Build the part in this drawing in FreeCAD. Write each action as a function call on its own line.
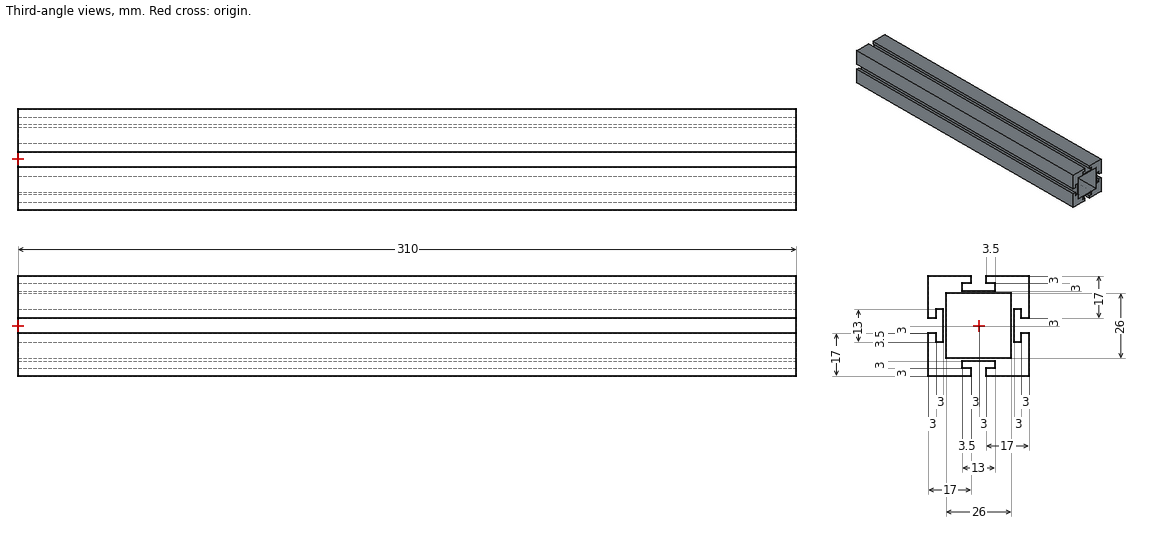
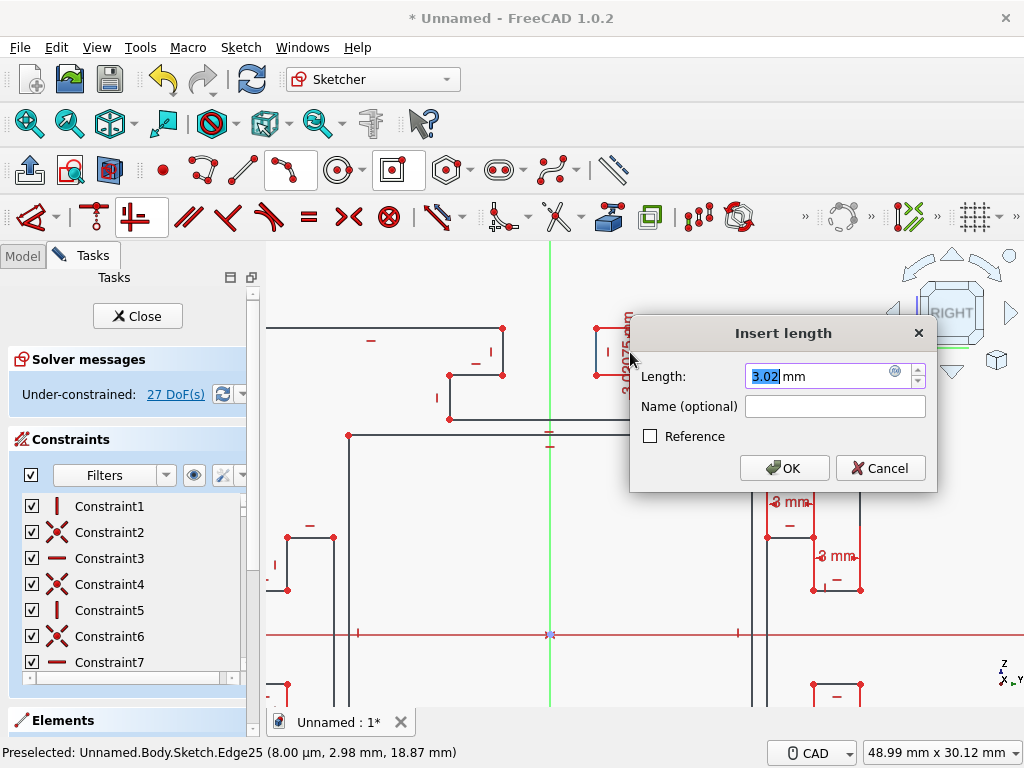
text(3)
key(Return)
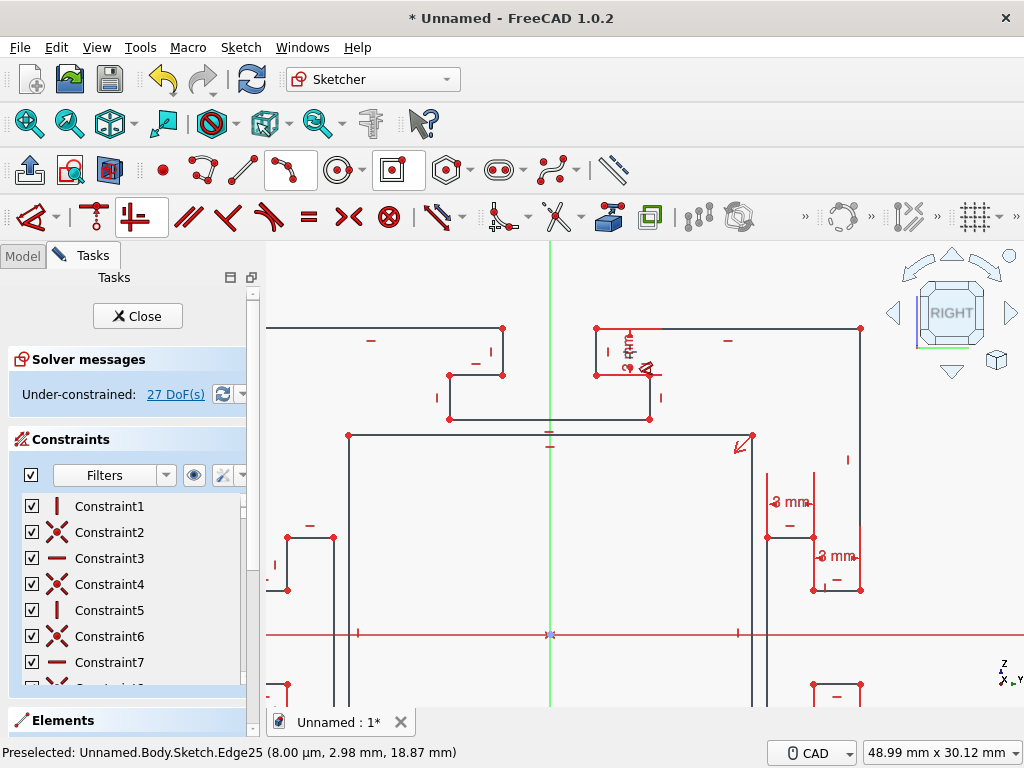
click(650, 388)
click(684, 397)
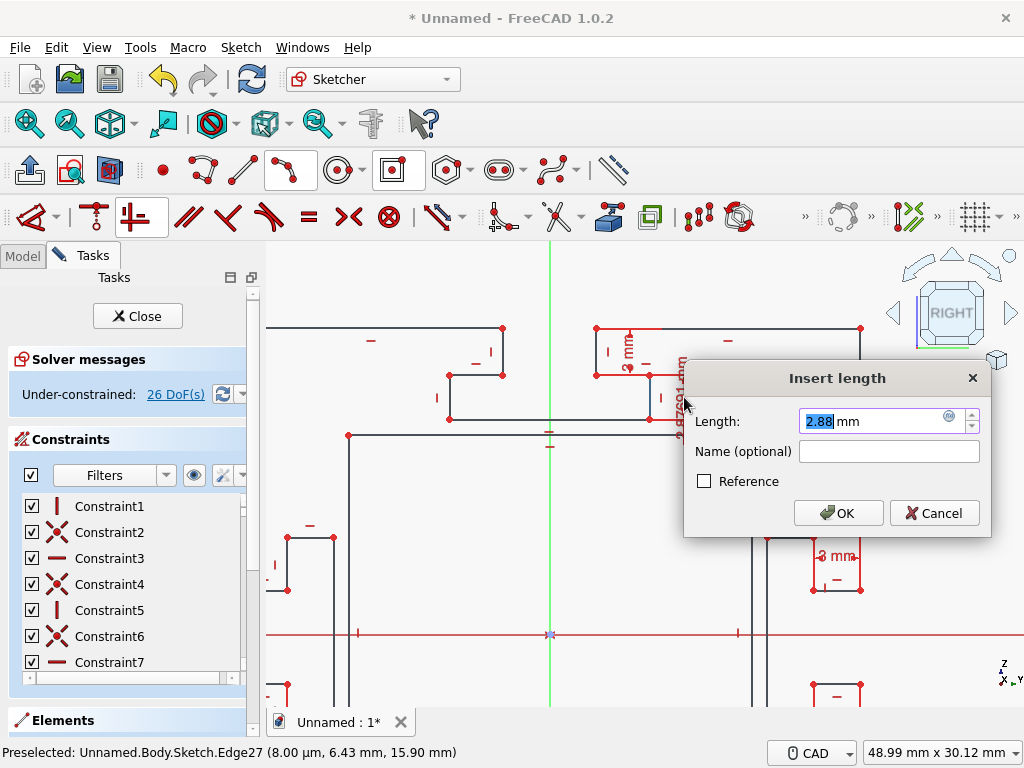
text(3)
key(Return)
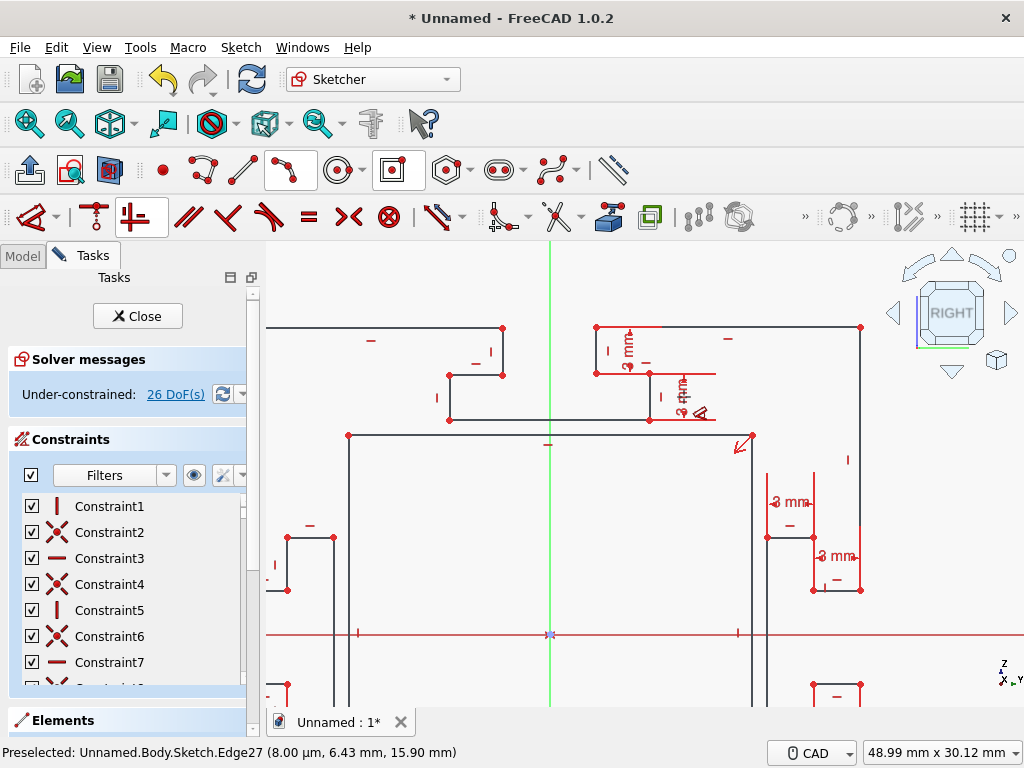
click(450, 407)
click(416, 398)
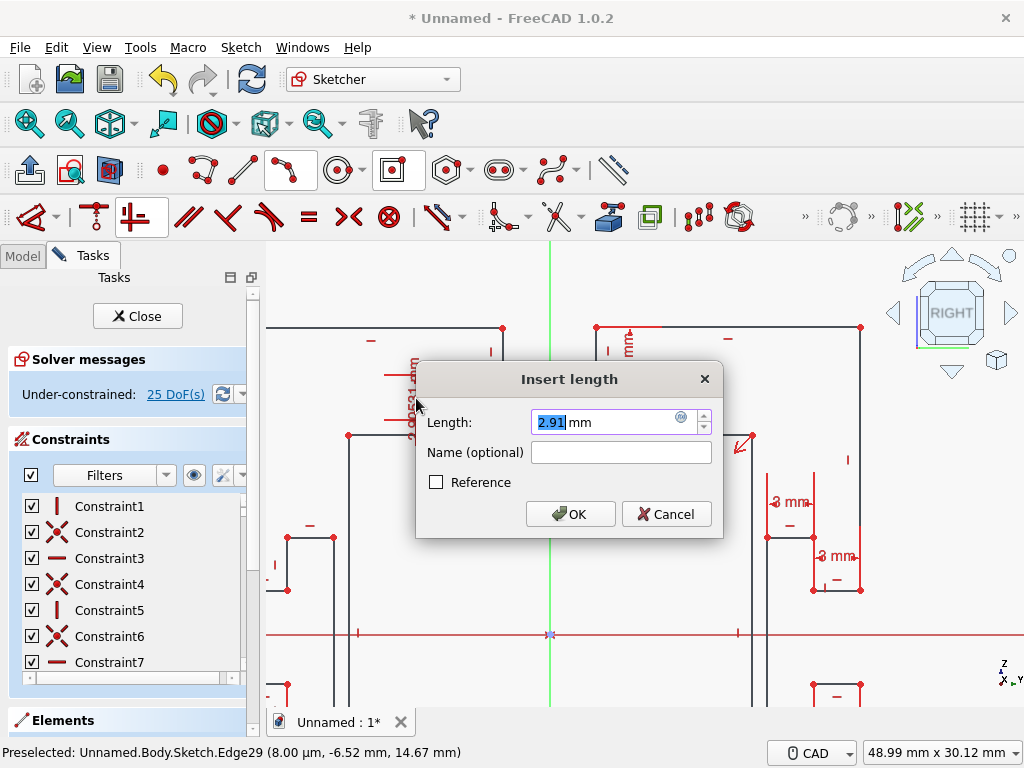
text(3)
key(Return)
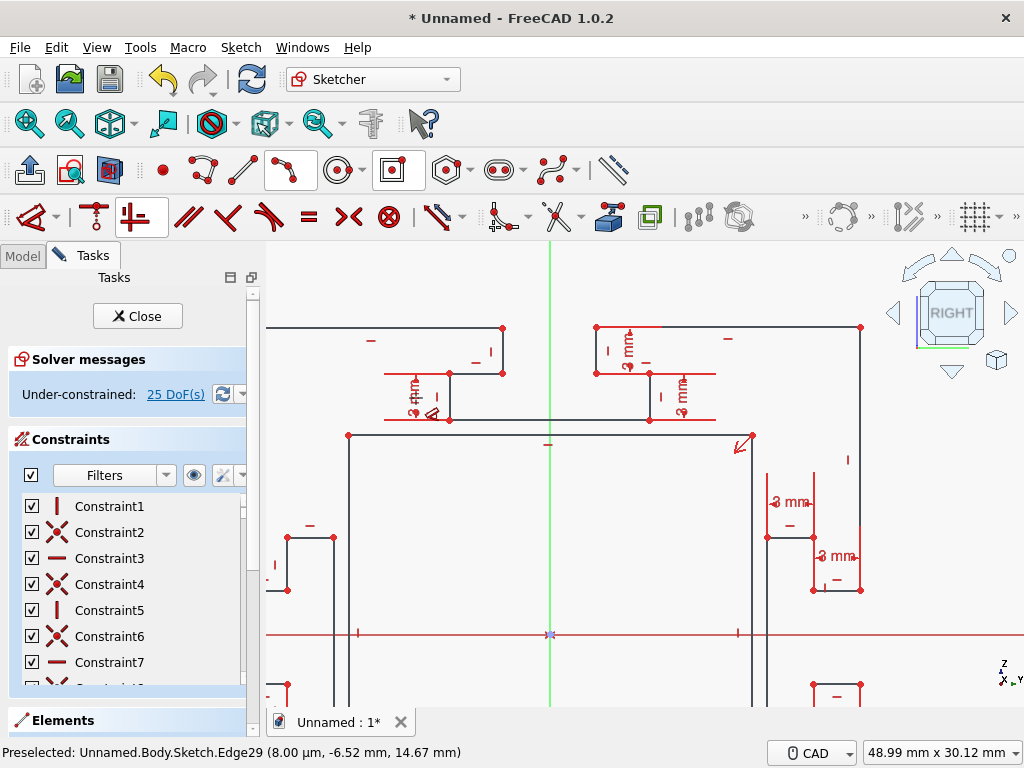
click(503, 360)
click(469, 351)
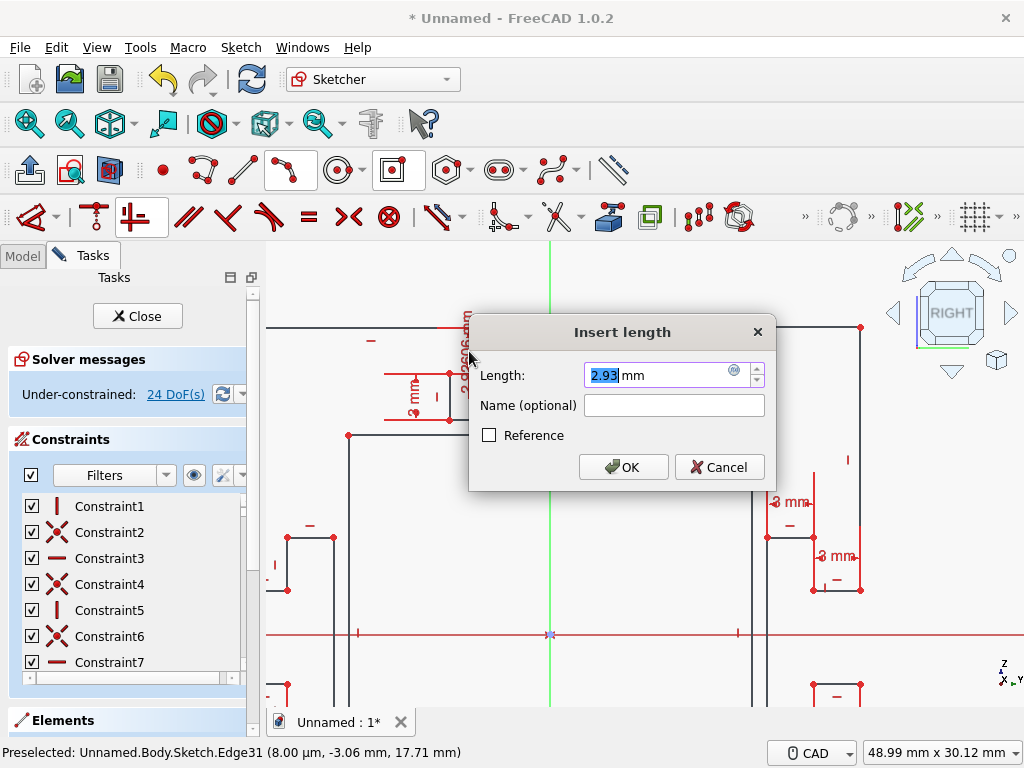
text(3)
key(Return)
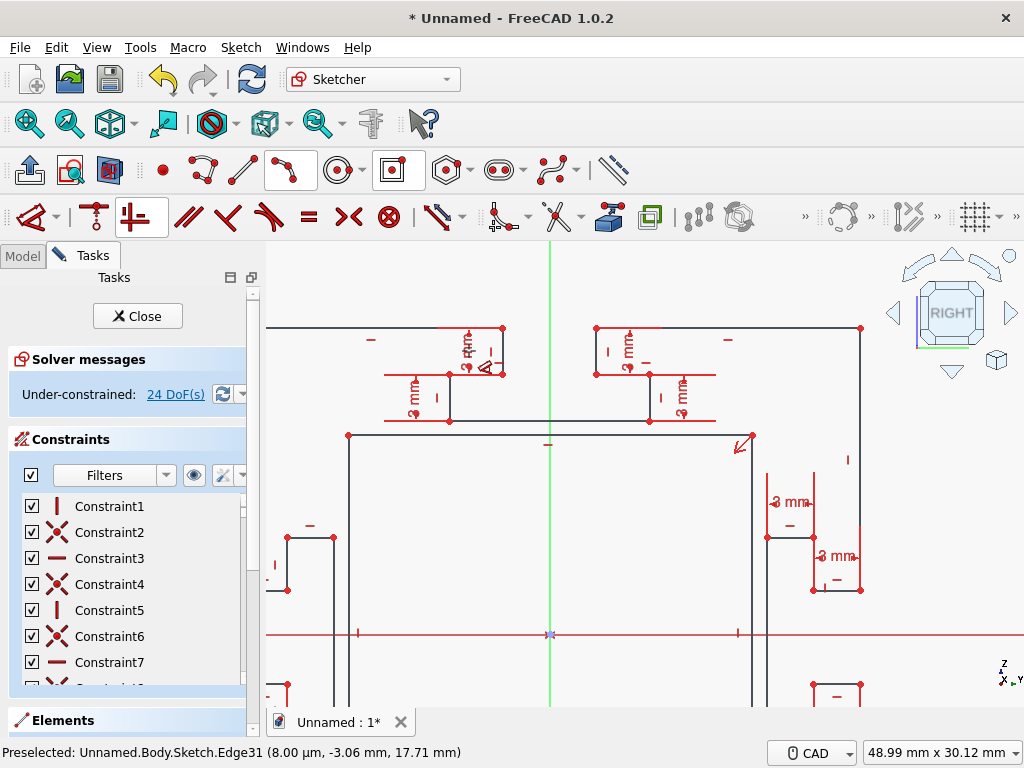
scroll(598, 343, down, 4)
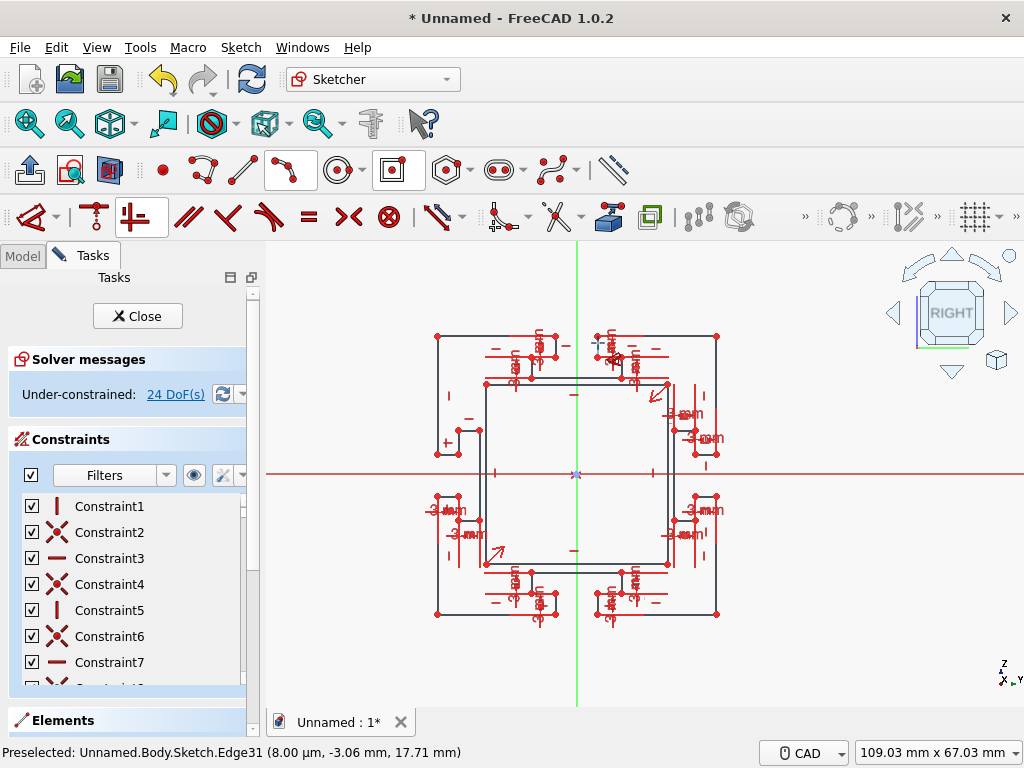
scroll(444, 455, up, 4)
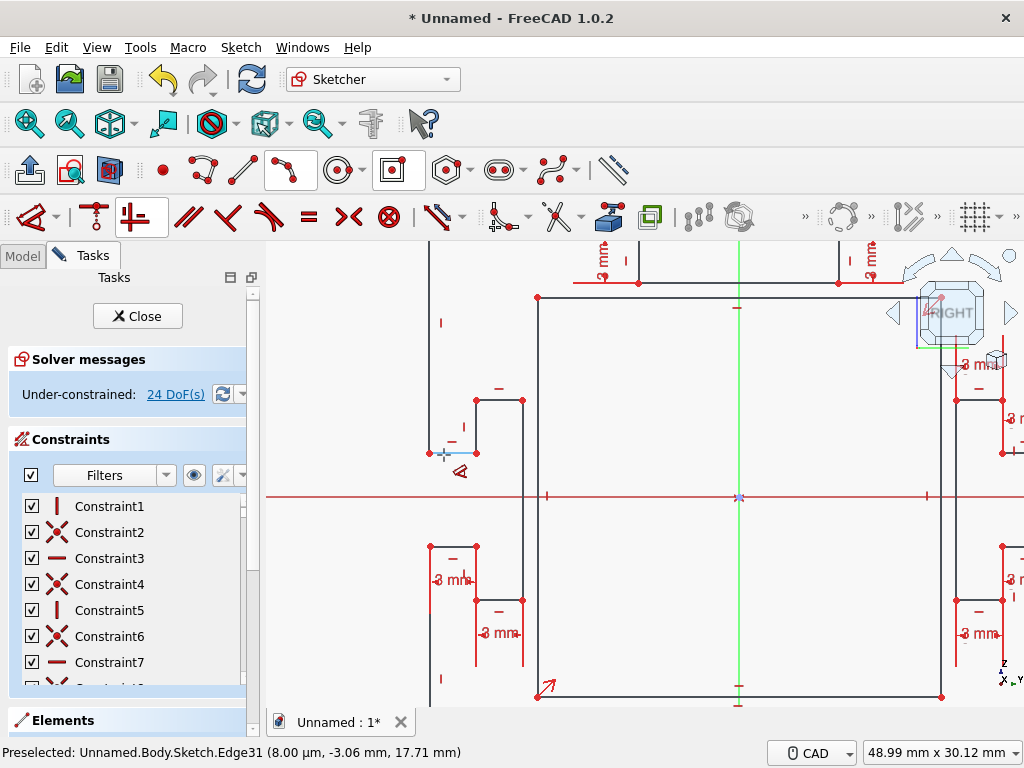
click(443, 453)
click(453, 419)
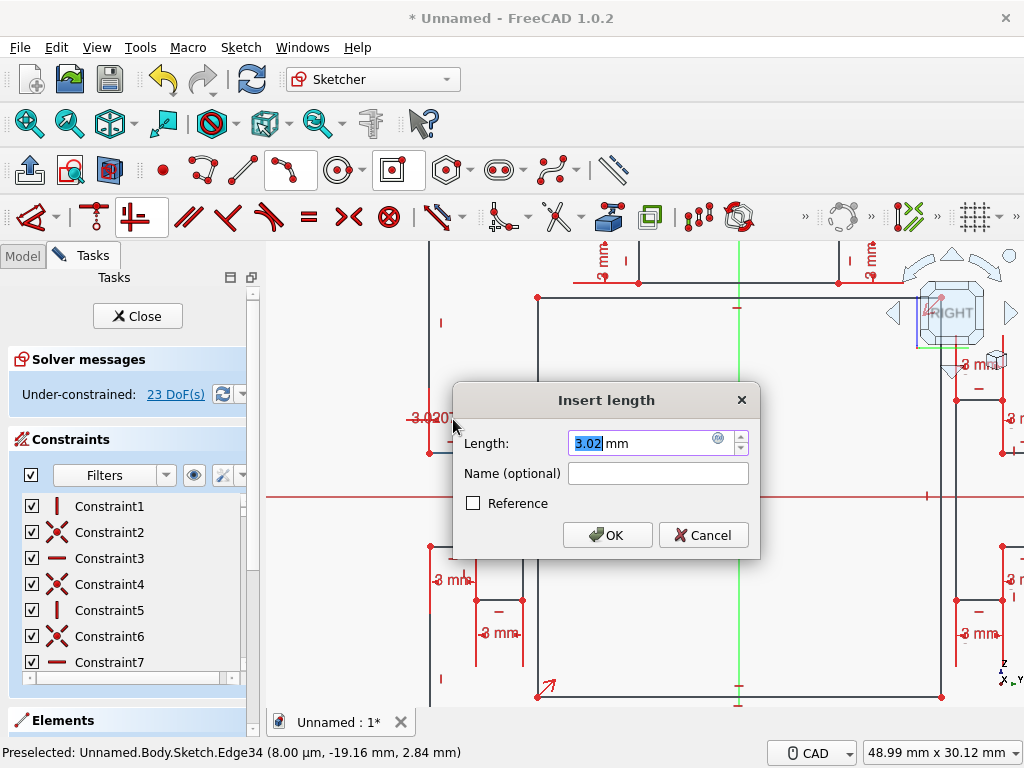
text(3)
key(Return)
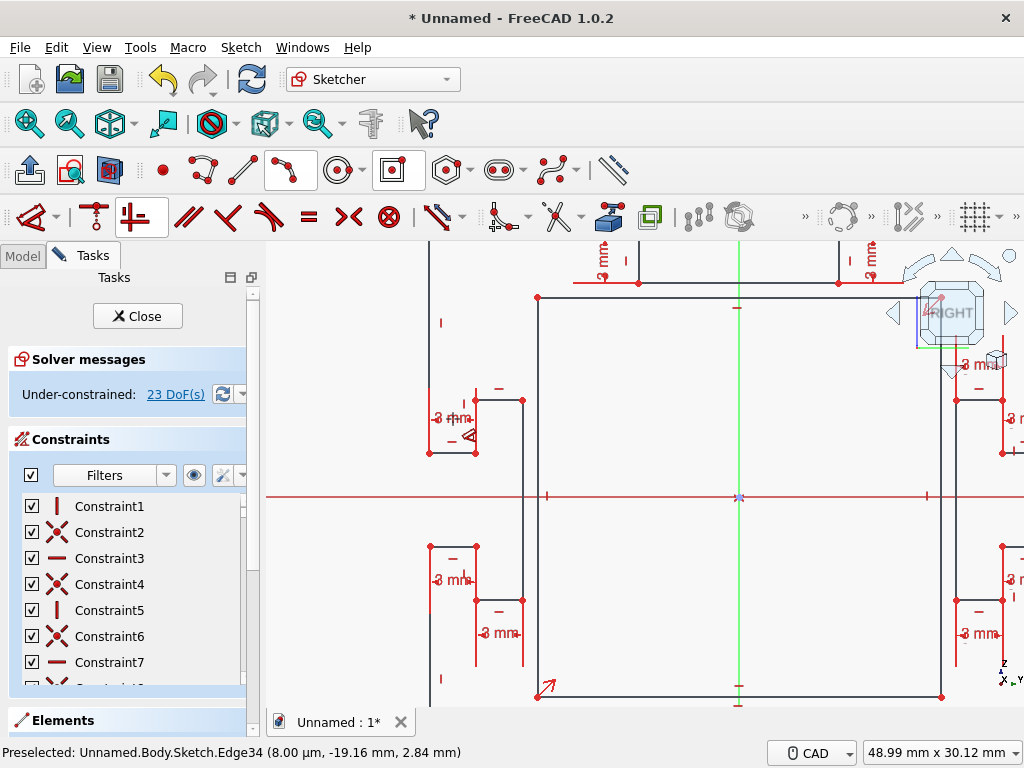
click(490, 400)
click(499, 366)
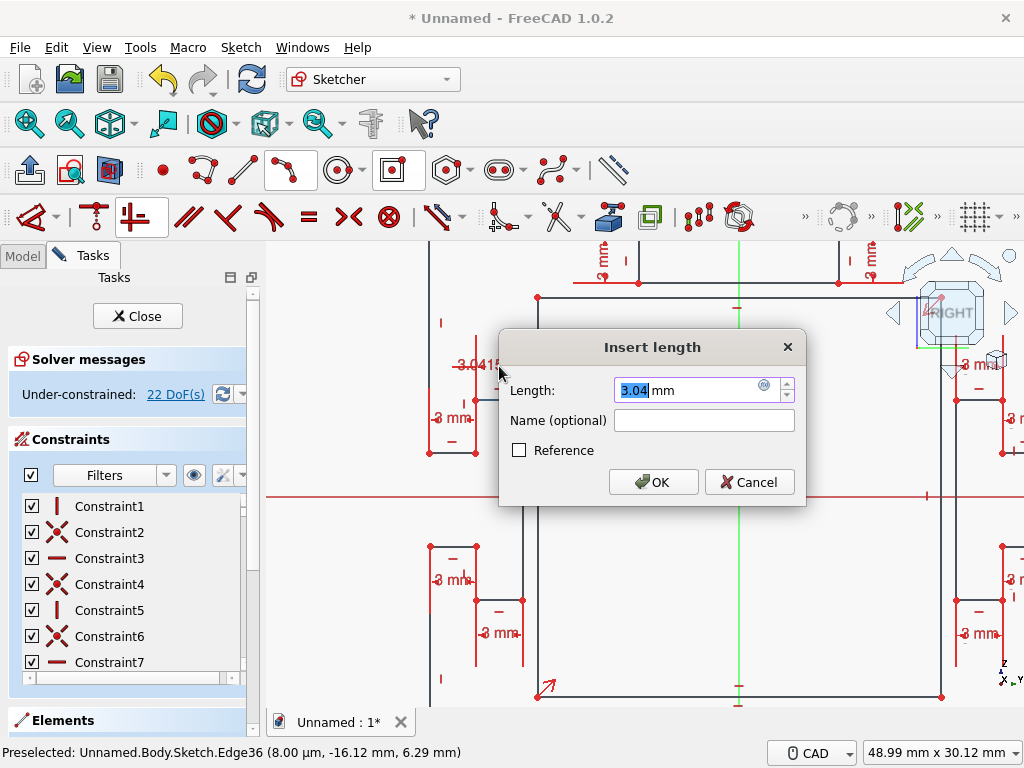
text(3)
key(Return)